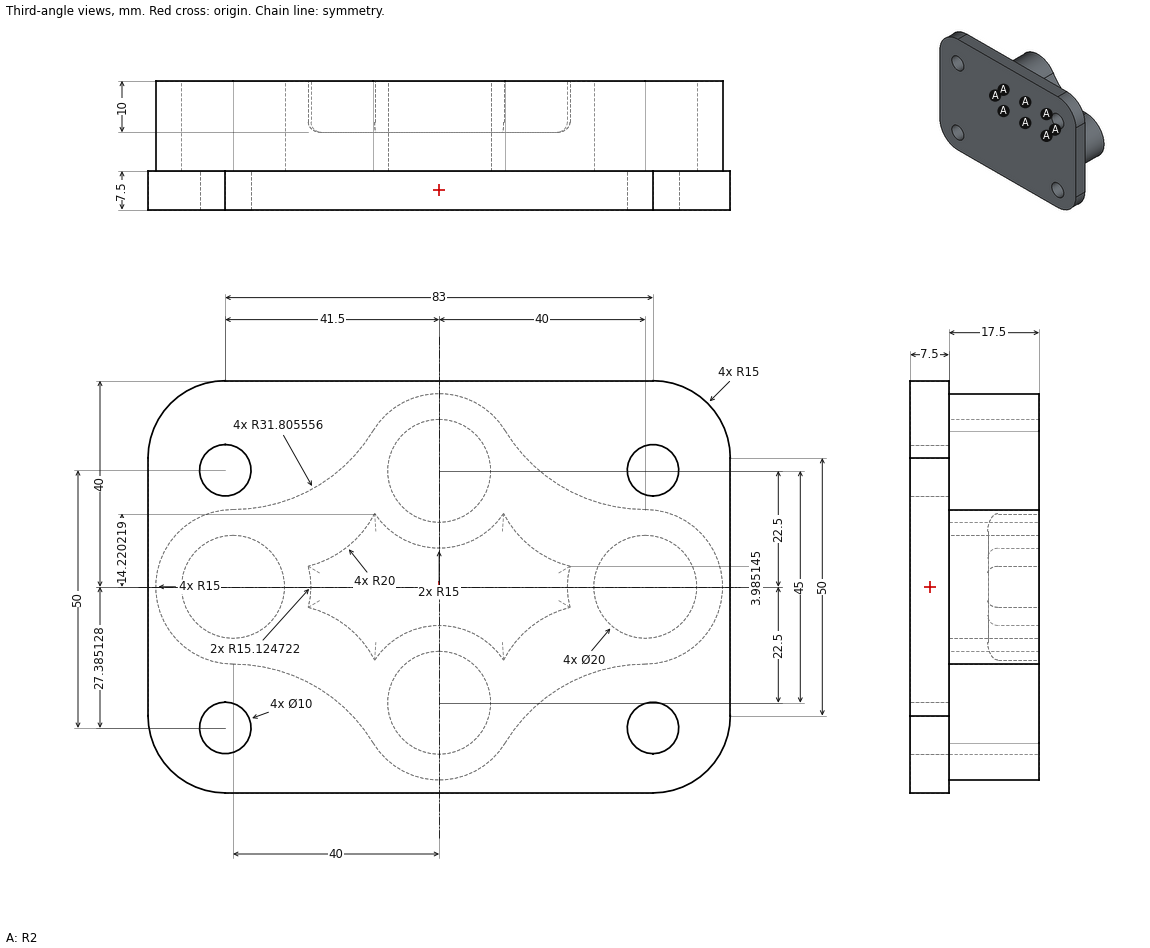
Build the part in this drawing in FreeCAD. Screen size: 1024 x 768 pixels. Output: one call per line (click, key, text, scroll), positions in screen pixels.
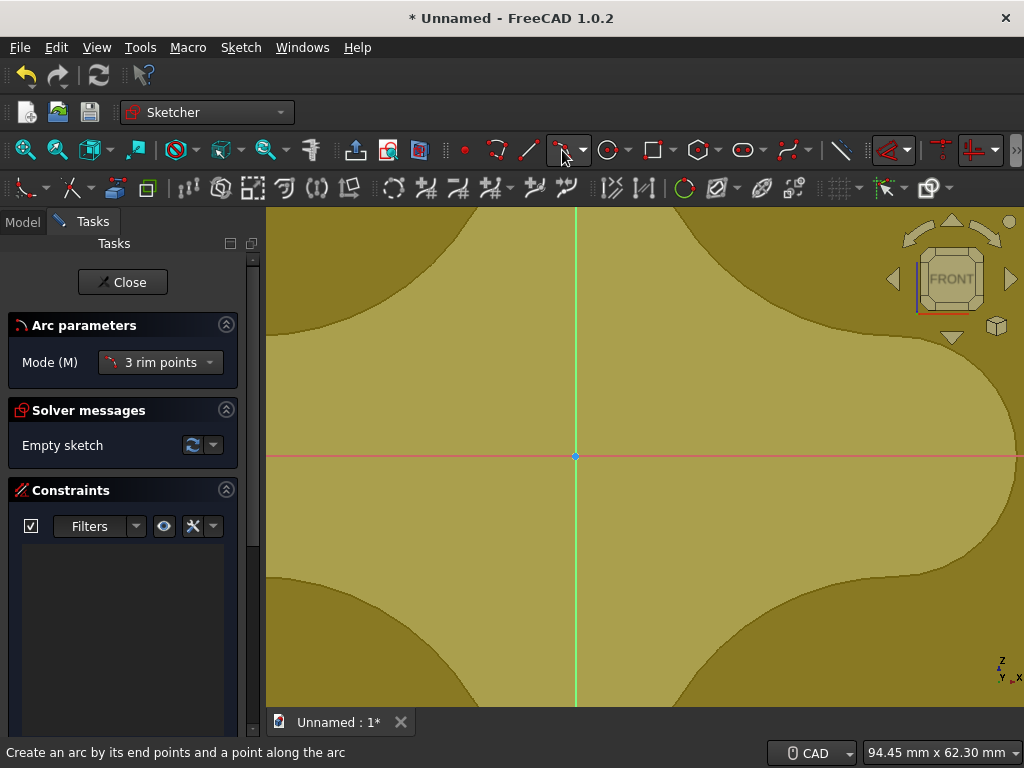
click(475, 342)
click(676, 342)
click(552, 394)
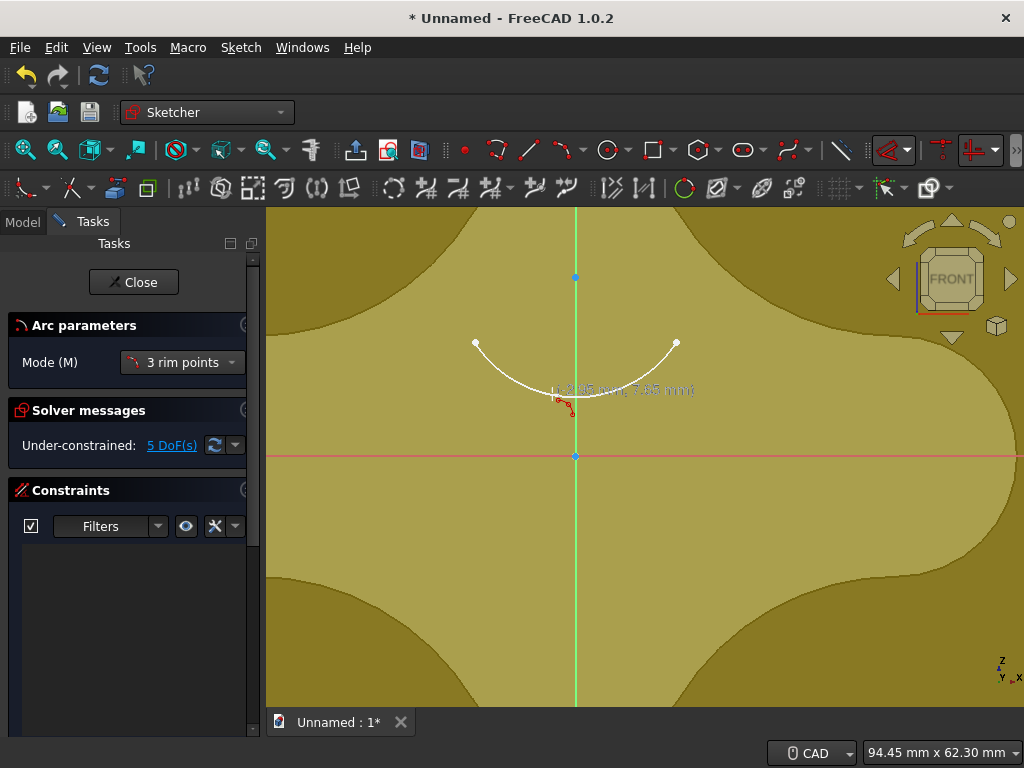
click(676, 343)
click(780, 424)
click(719, 394)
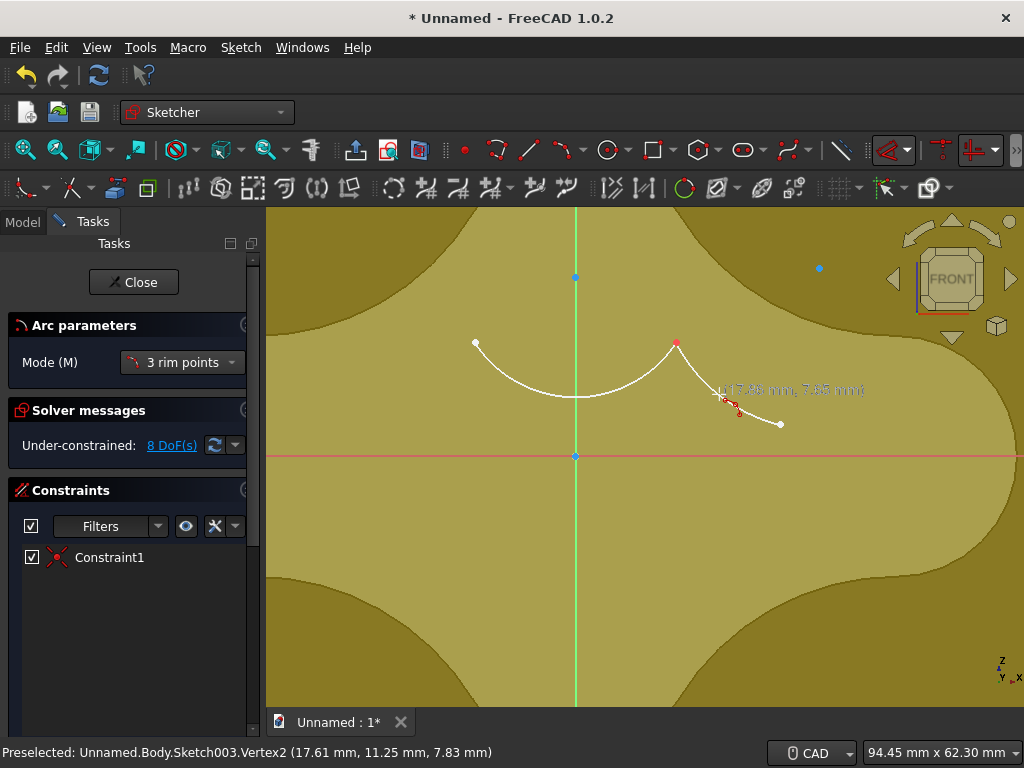
click(780, 425)
click(780, 488)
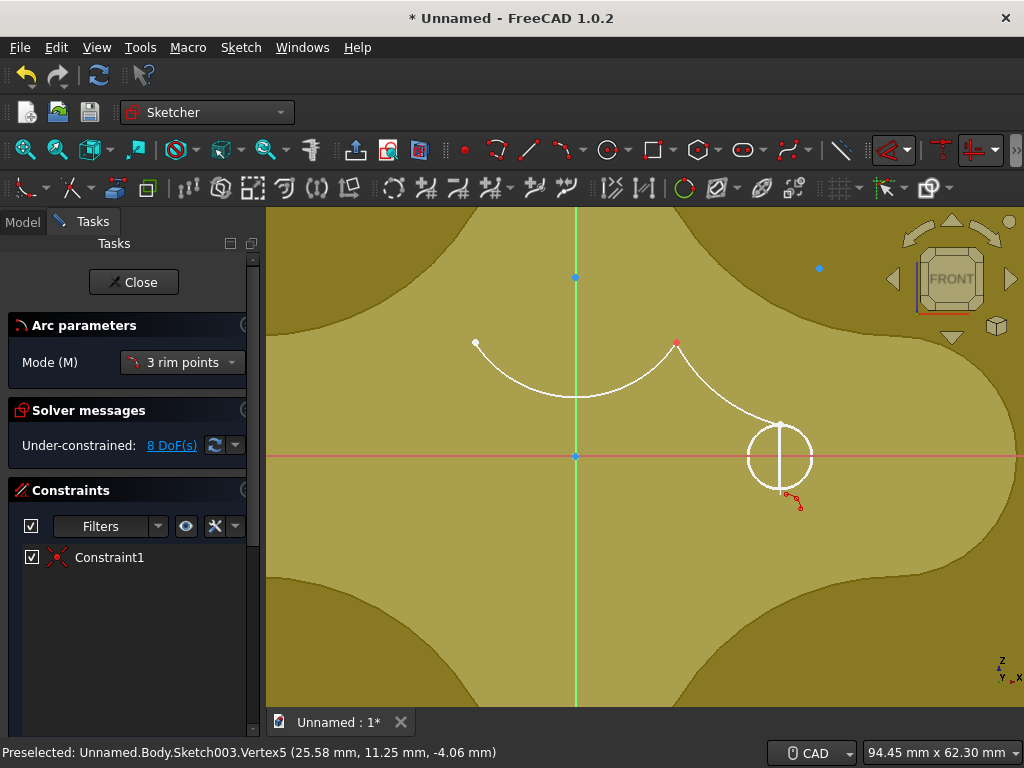
scroll(775, 450, up, 7)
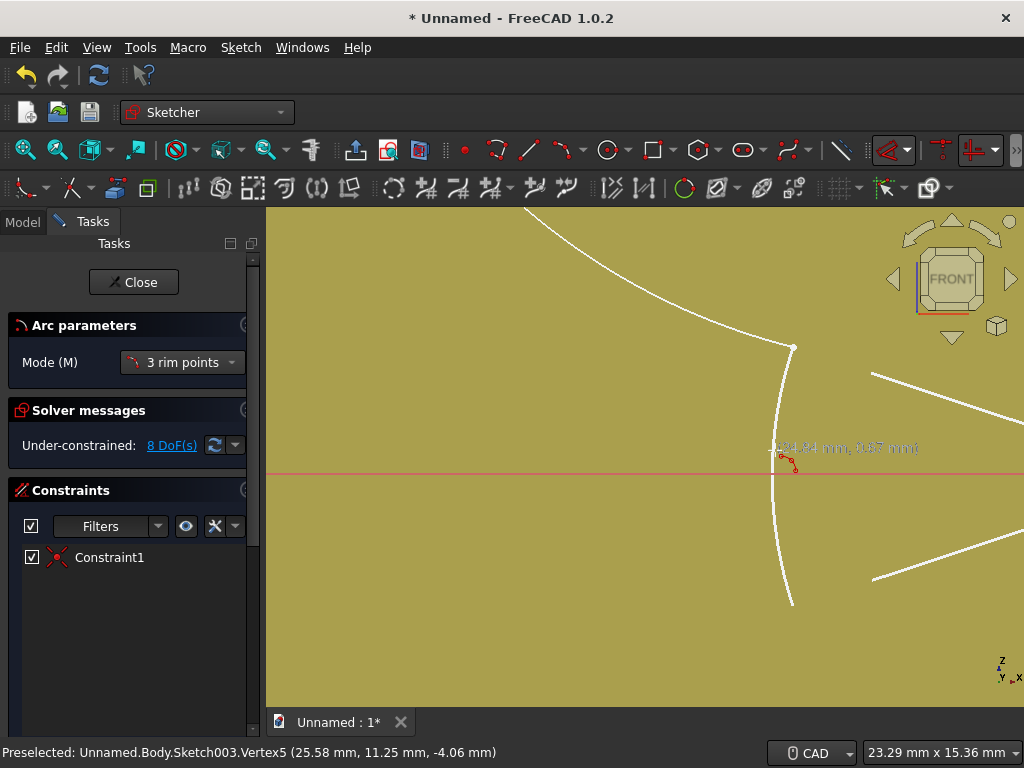
click(775, 448)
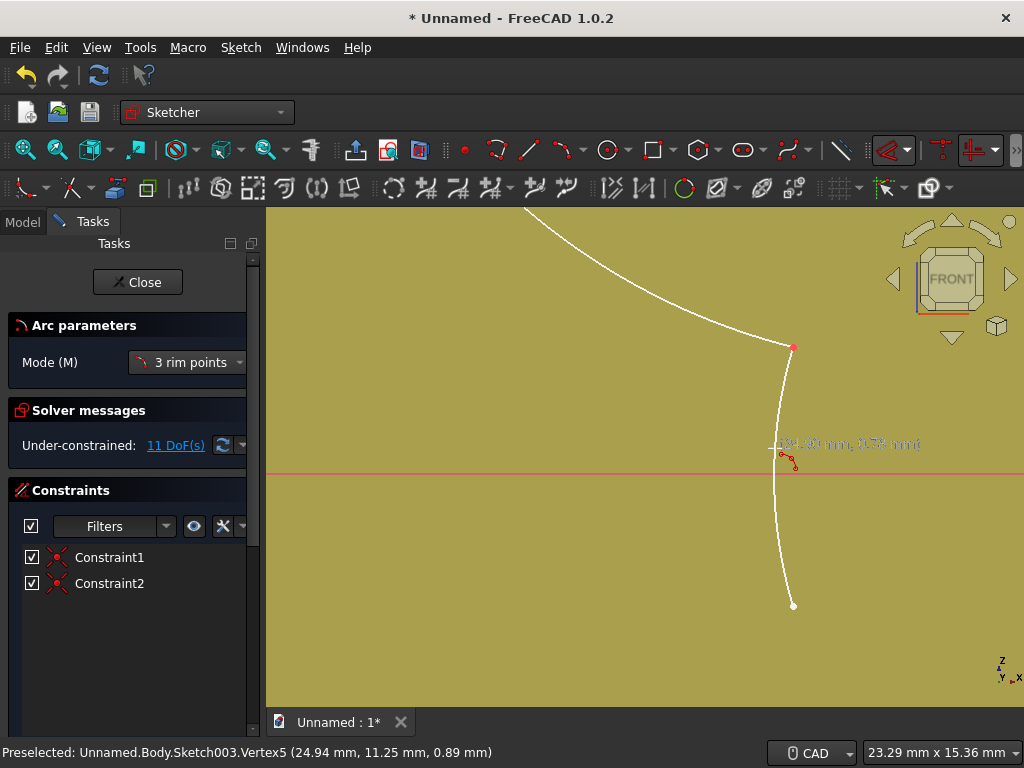
scroll(777, 451, down, 7)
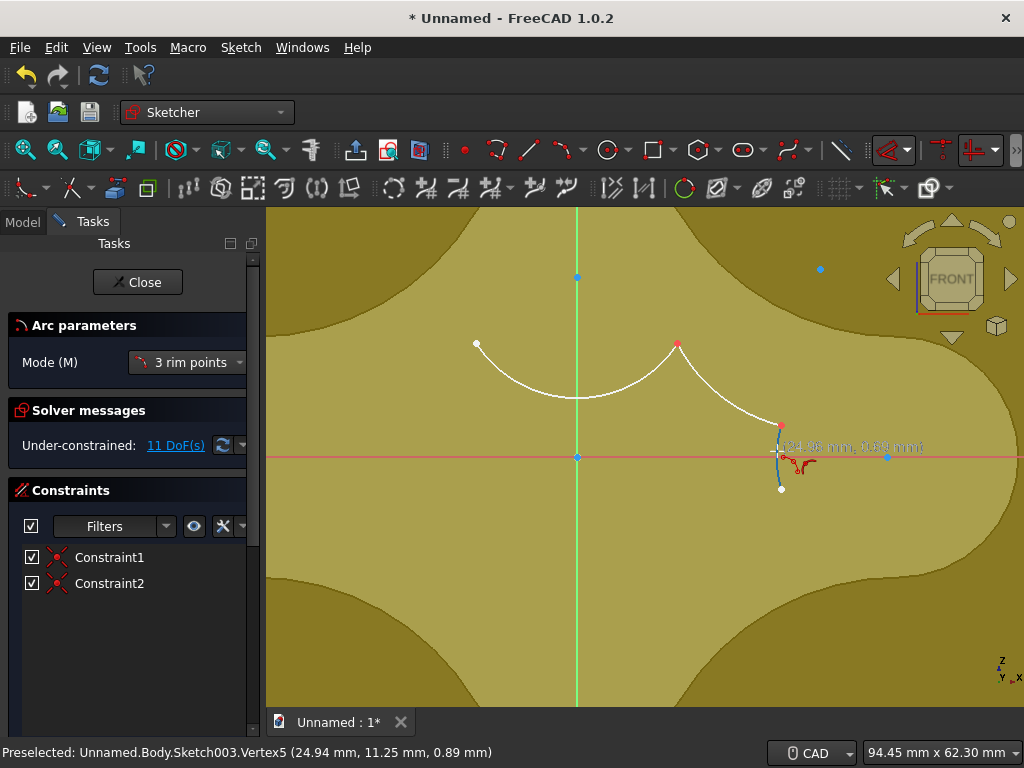
click(782, 490)
click(678, 571)
click(720, 519)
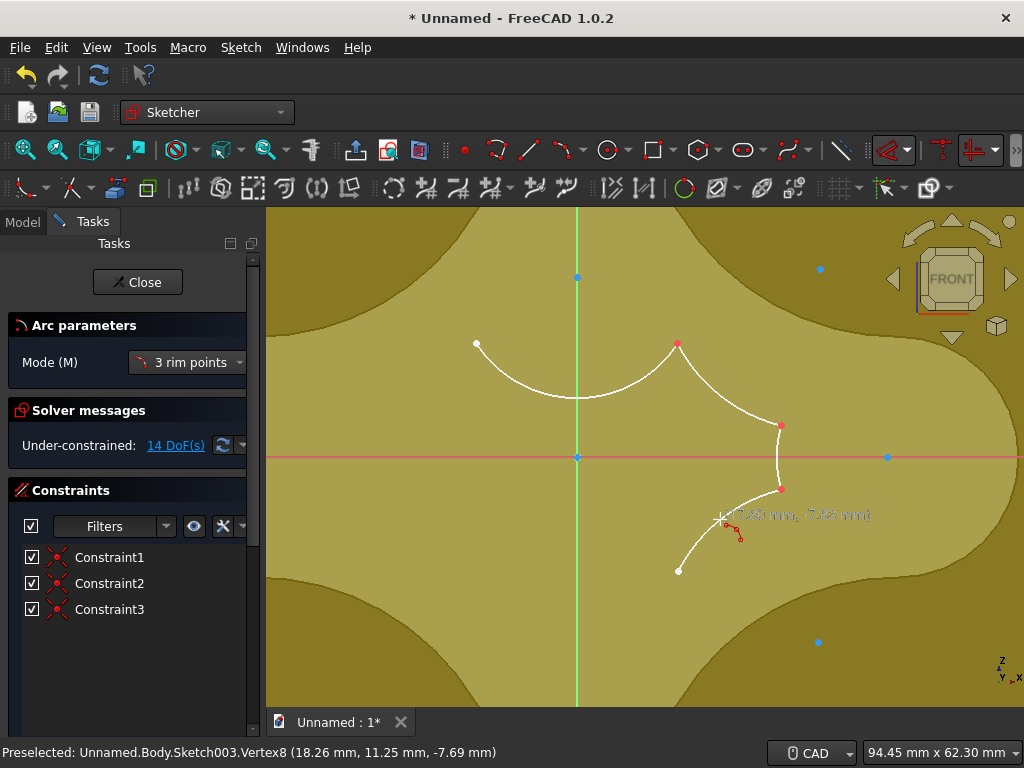
click(678, 572)
click(477, 571)
click(601, 520)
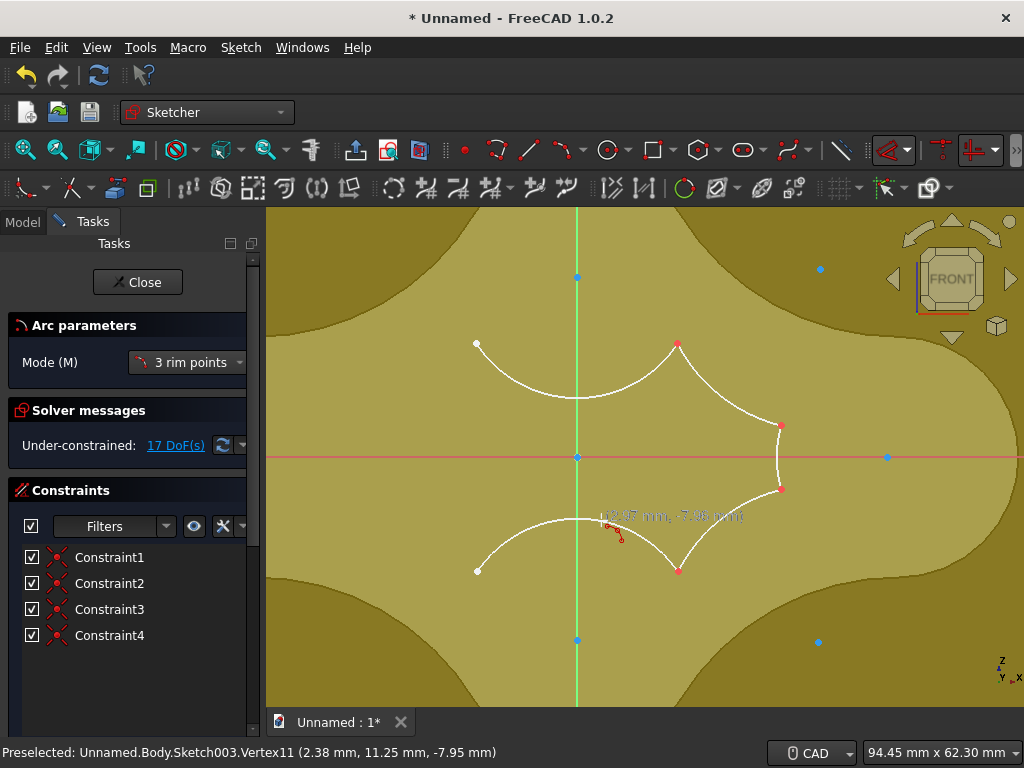
click(477, 572)
click(373, 489)
click(434, 519)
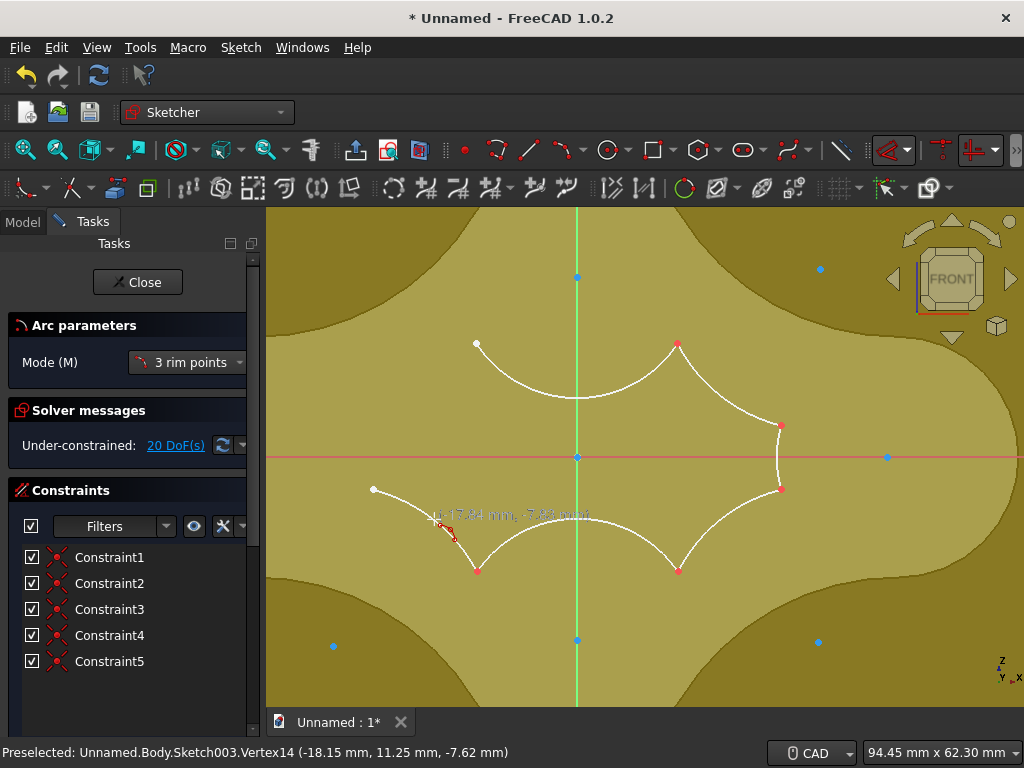
click(373, 490)
click(373, 425)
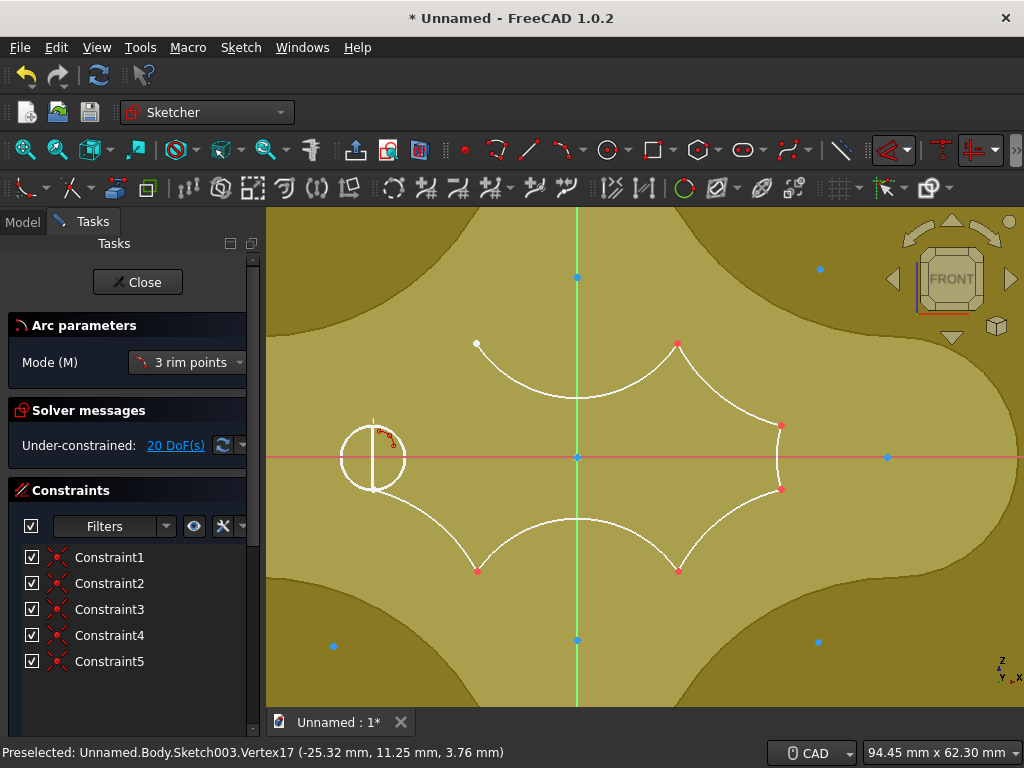
scroll(377, 464, up, 7)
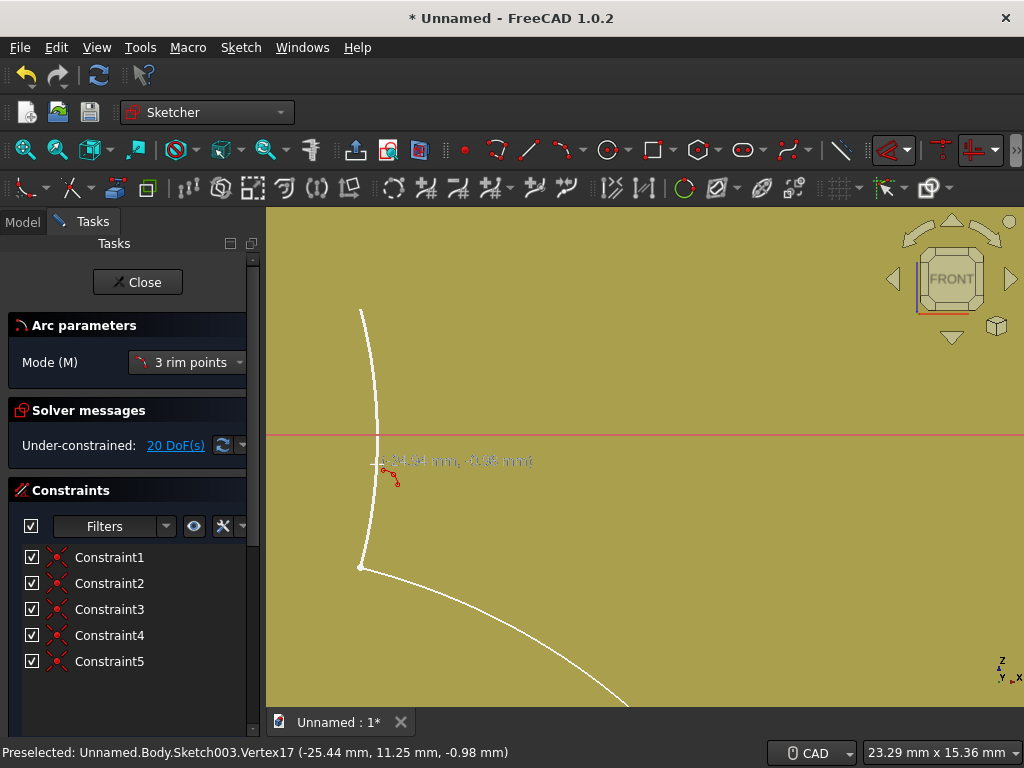
click(378, 461)